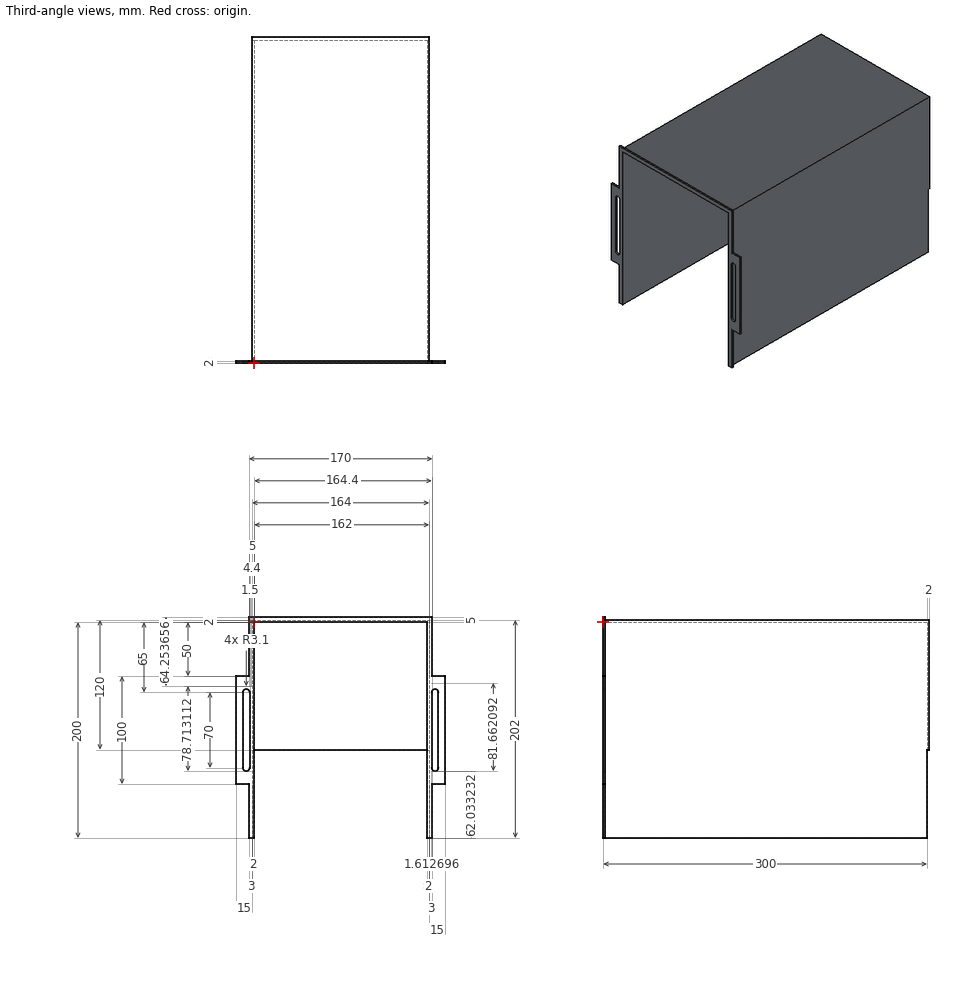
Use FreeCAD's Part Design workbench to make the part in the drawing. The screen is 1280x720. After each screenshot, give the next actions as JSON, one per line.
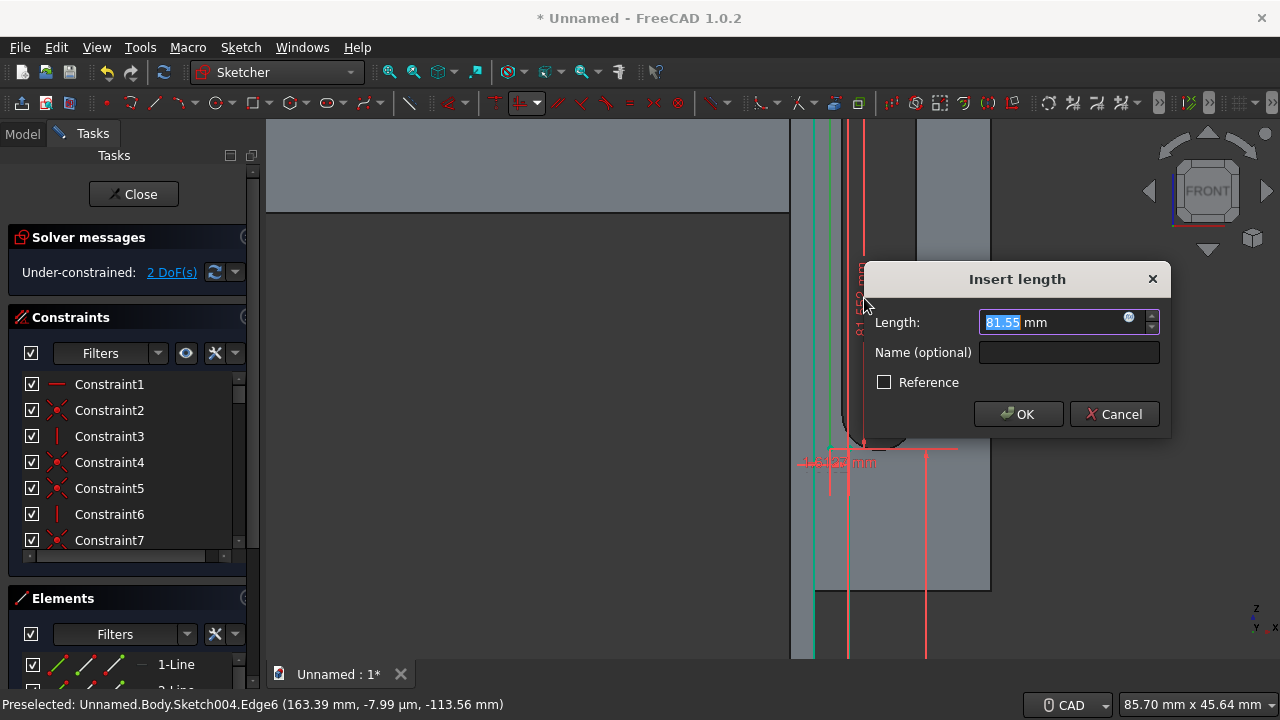
{"action": "type", "text": "81.662092"}
{"action": "key", "text": "Return"}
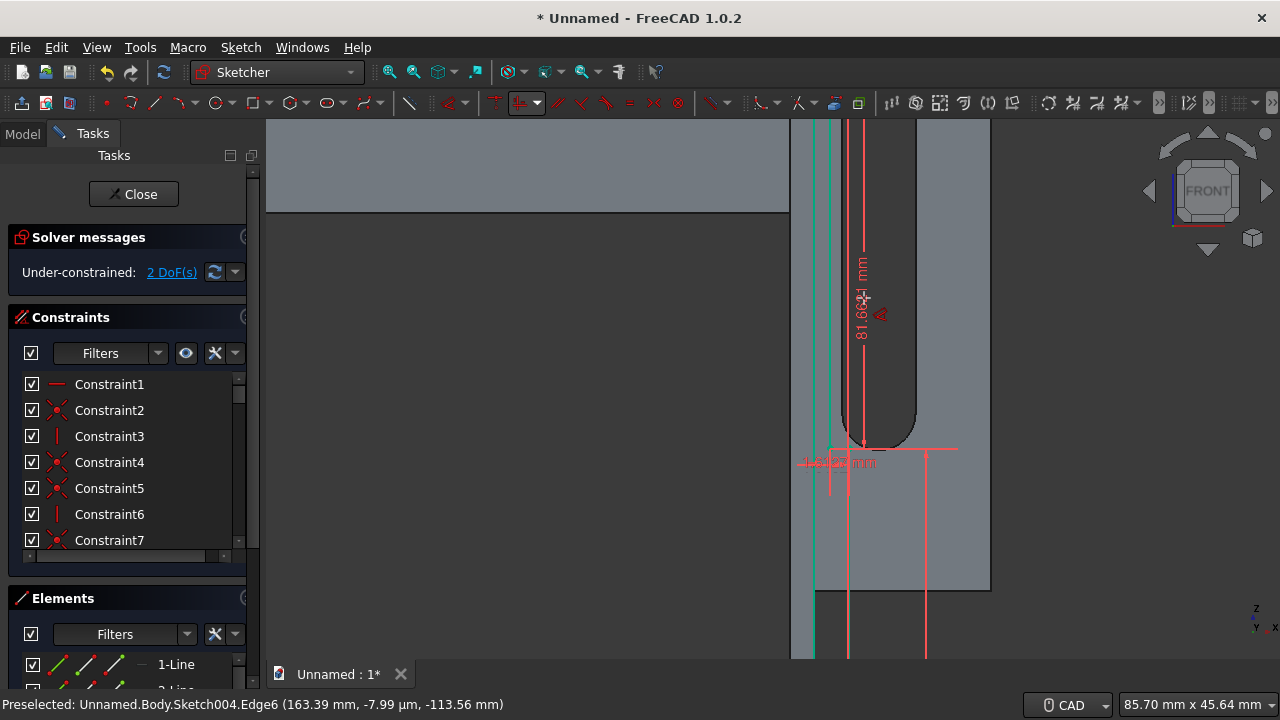
{"action": "scroll", "coordinate": [839, 455], "scroll_direction": "down", "scroll_amount": 10}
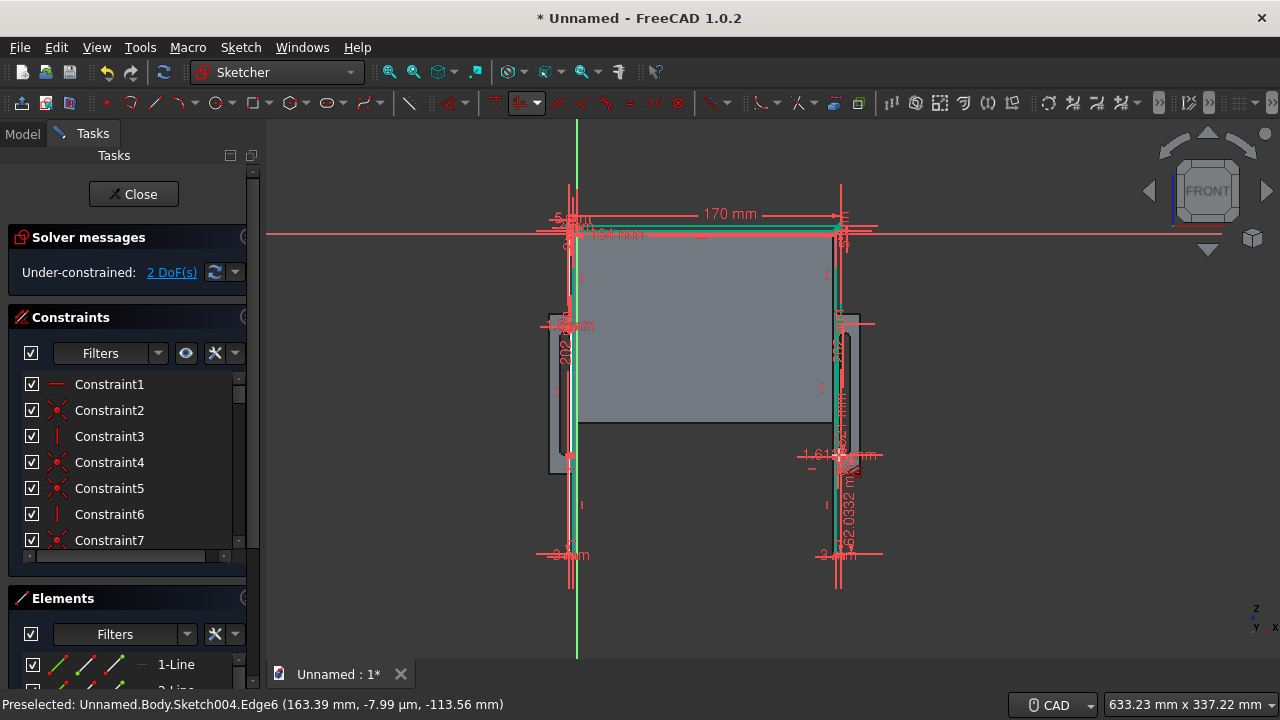
{"action": "scroll", "coordinate": [569, 257], "scroll_direction": "up", "scroll_amount": 6}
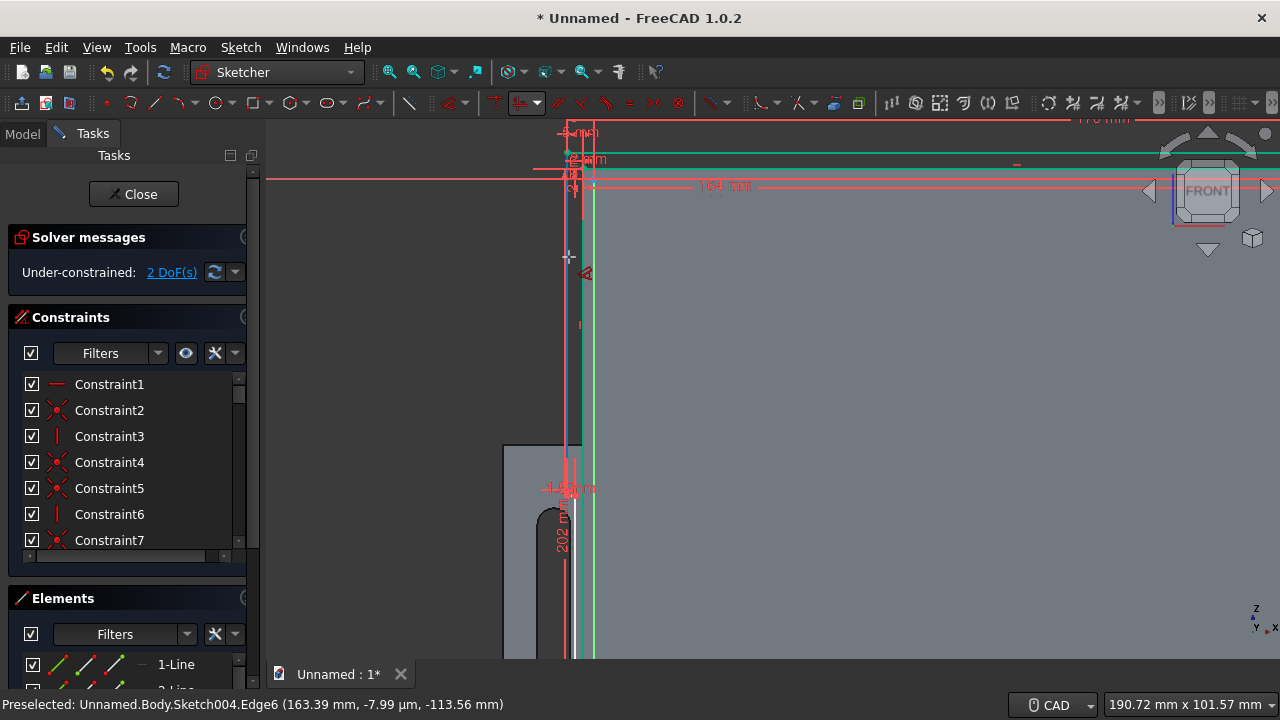
{"action": "left_click", "coordinate": [567, 256]}
{"action": "left_click", "coordinate": [533, 324]}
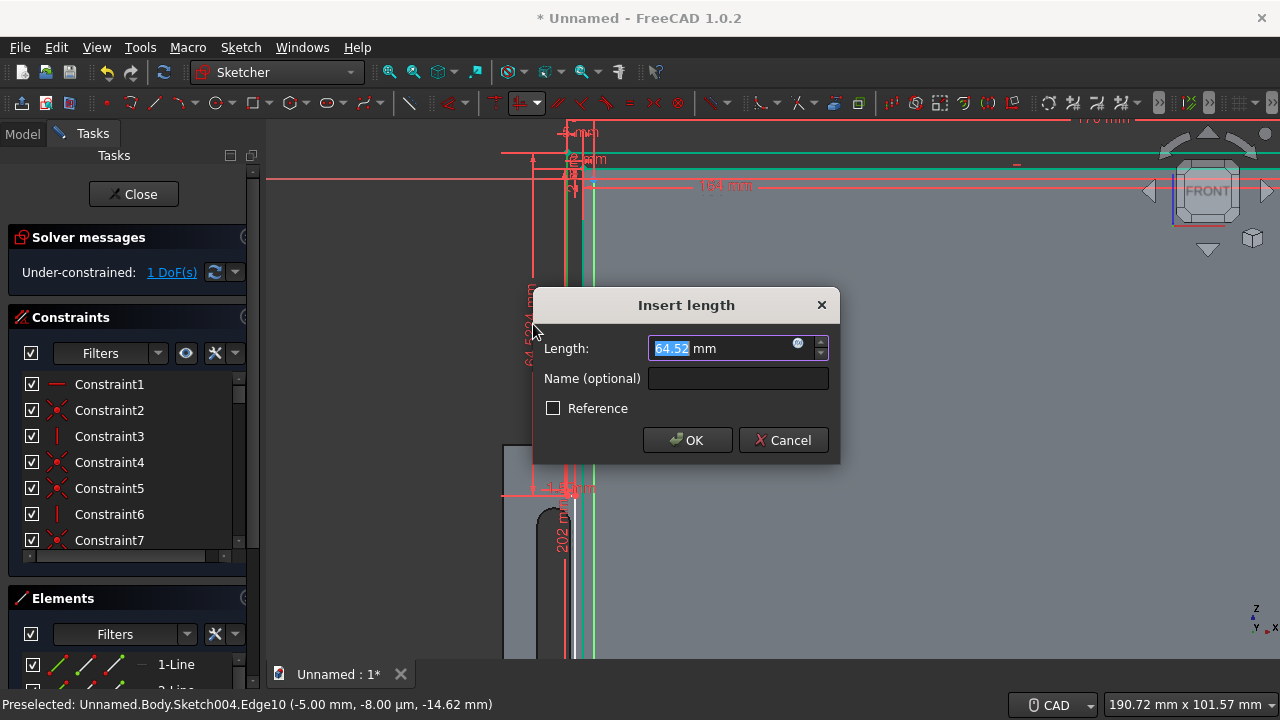
{"action": "type", "text": "64.253656"}
{"action": "key", "text": "Return"}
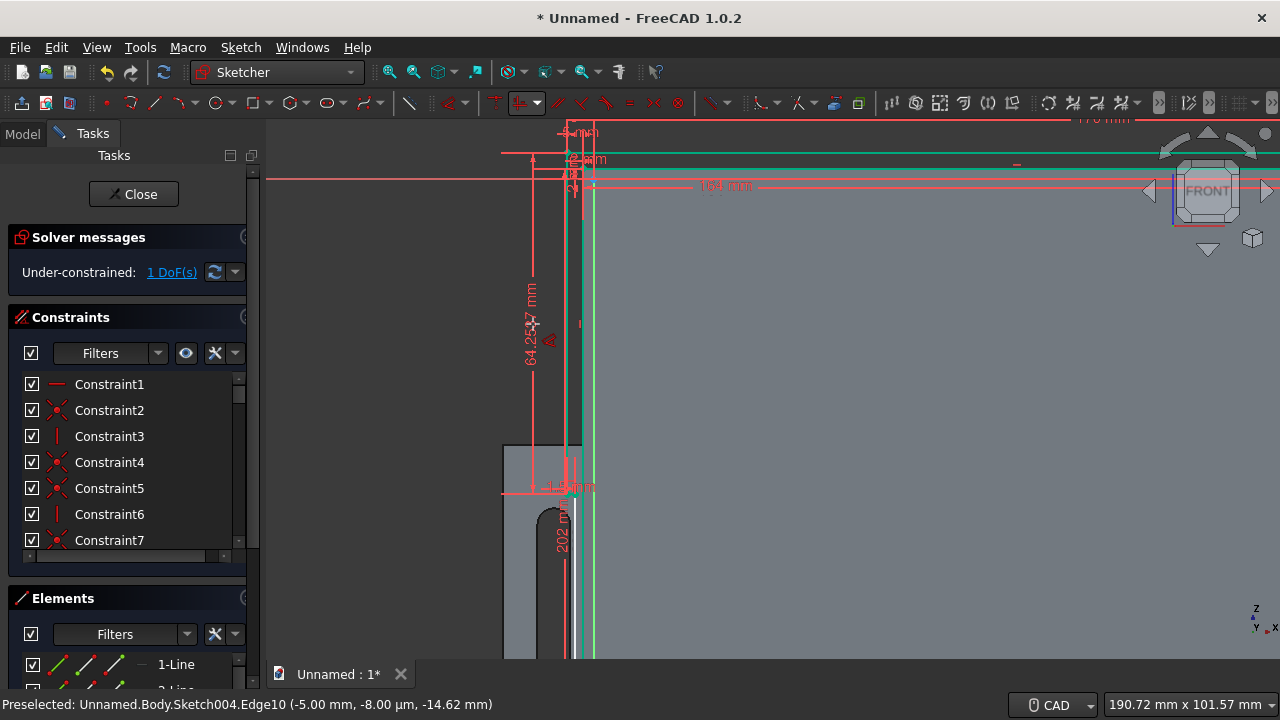
{"action": "scroll", "coordinate": [575, 620], "scroll_direction": "up", "scroll_amount": 3}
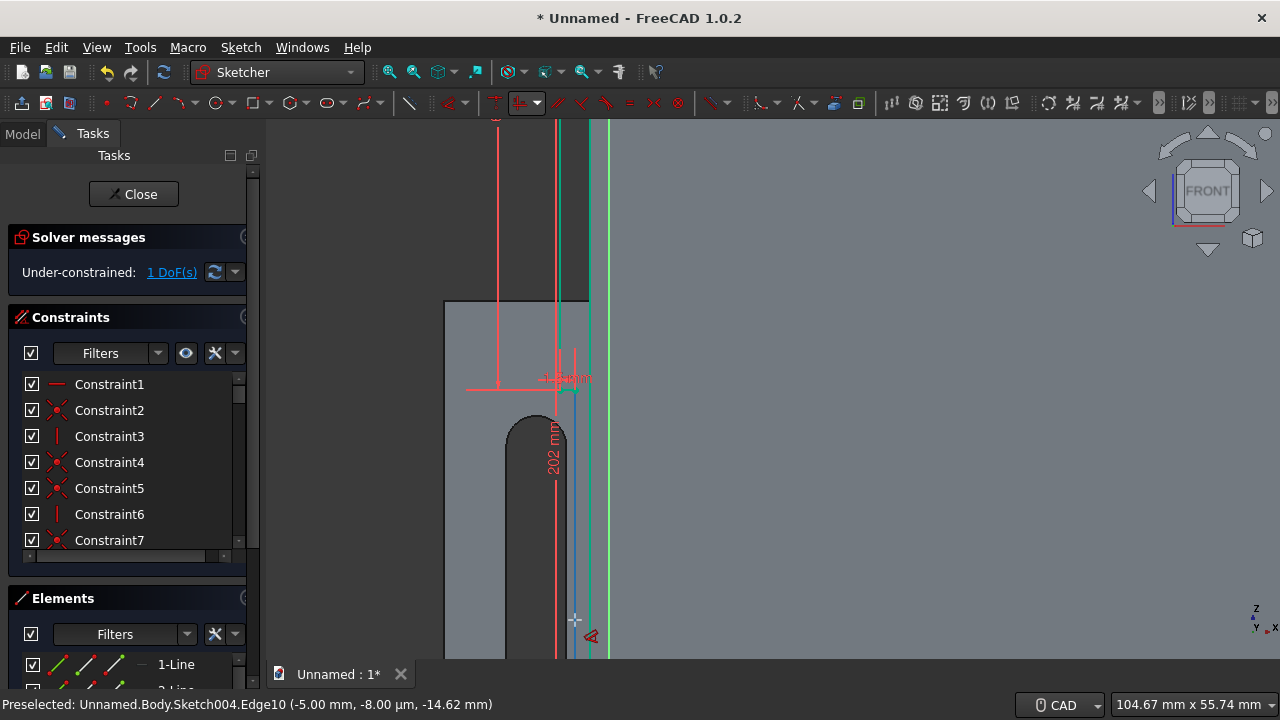
{"action": "left_click", "coordinate": [575, 620]}
{"action": "left_click", "coordinate": [541, 511]}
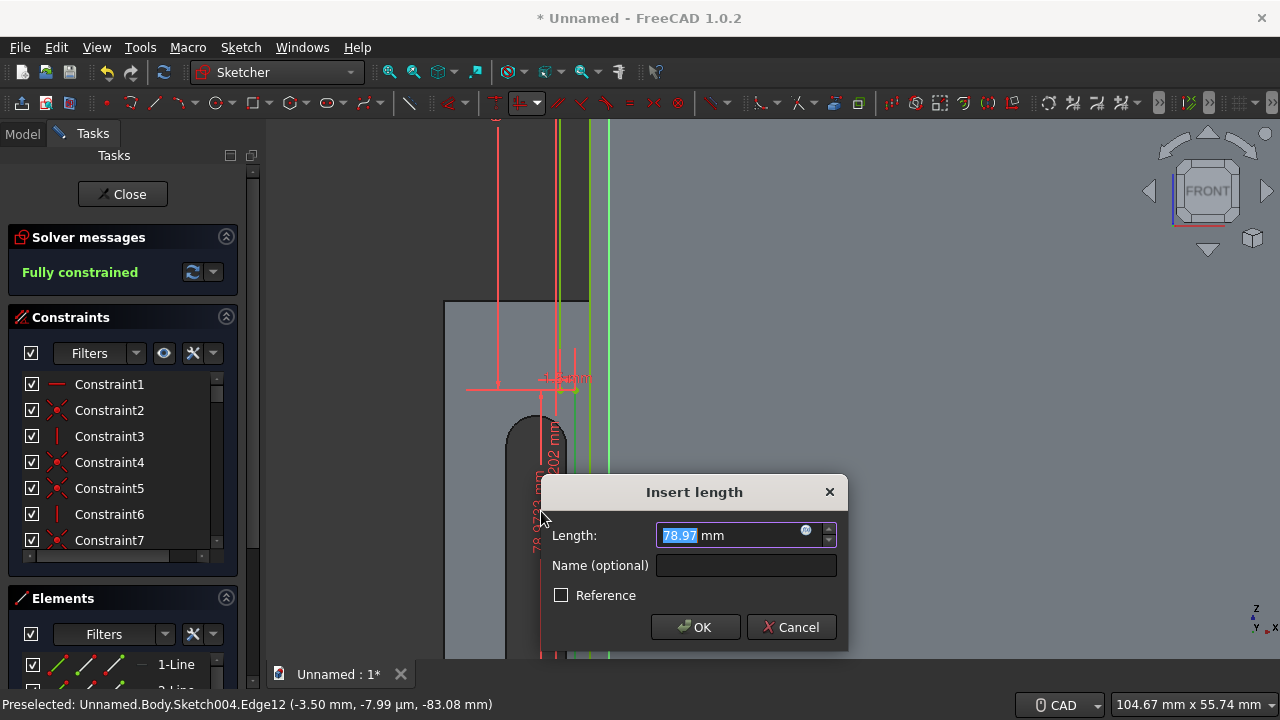
{"action": "type", "text": "78.713112"}
{"action": "key", "text": "Return"}
{"action": "key", "text": "Escape"}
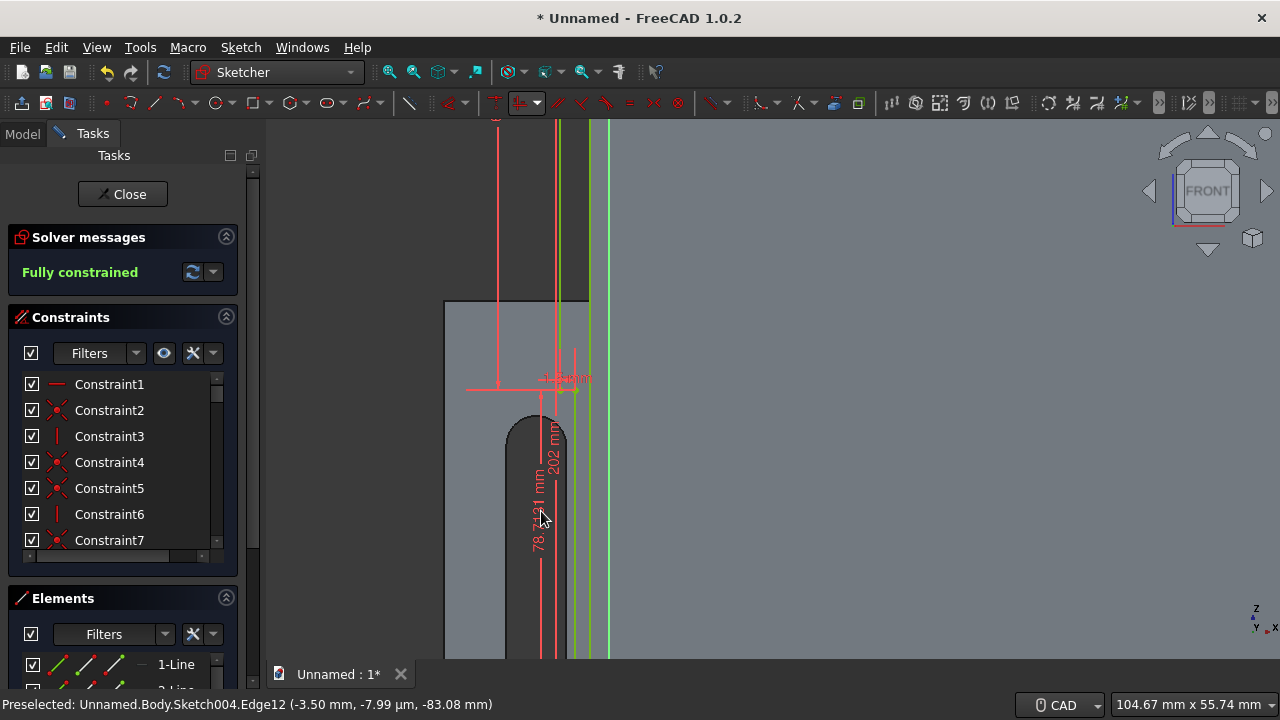
{"action": "left_click", "coordinate": [123, 194]}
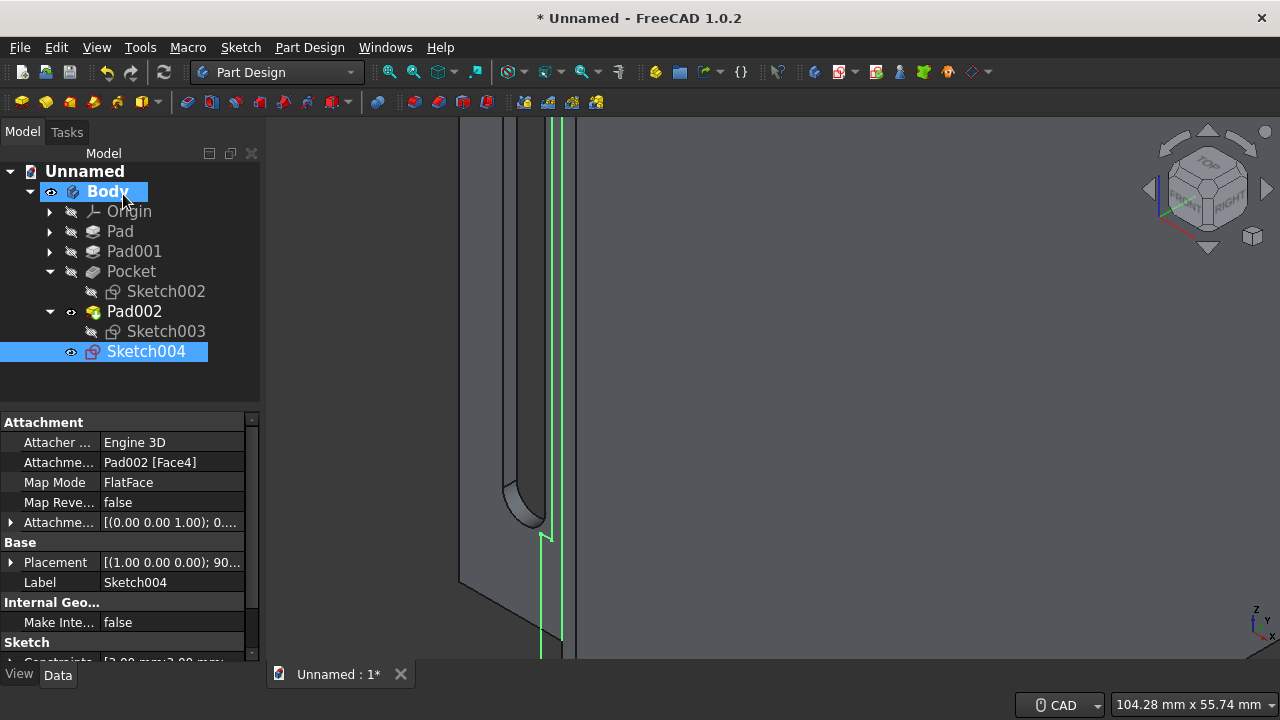
{"action": "left_click", "coordinate": [22, 102]}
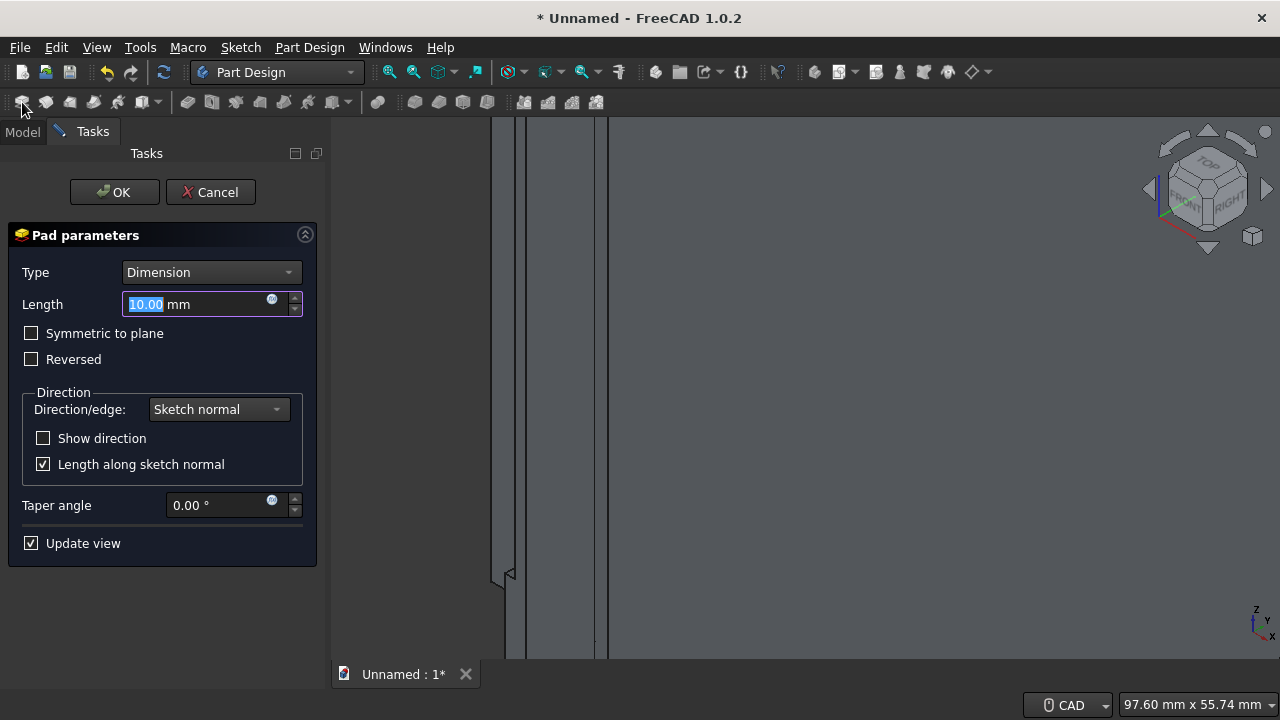
{"action": "type", "text": "2"}
{"action": "key", "text": "Tab"}